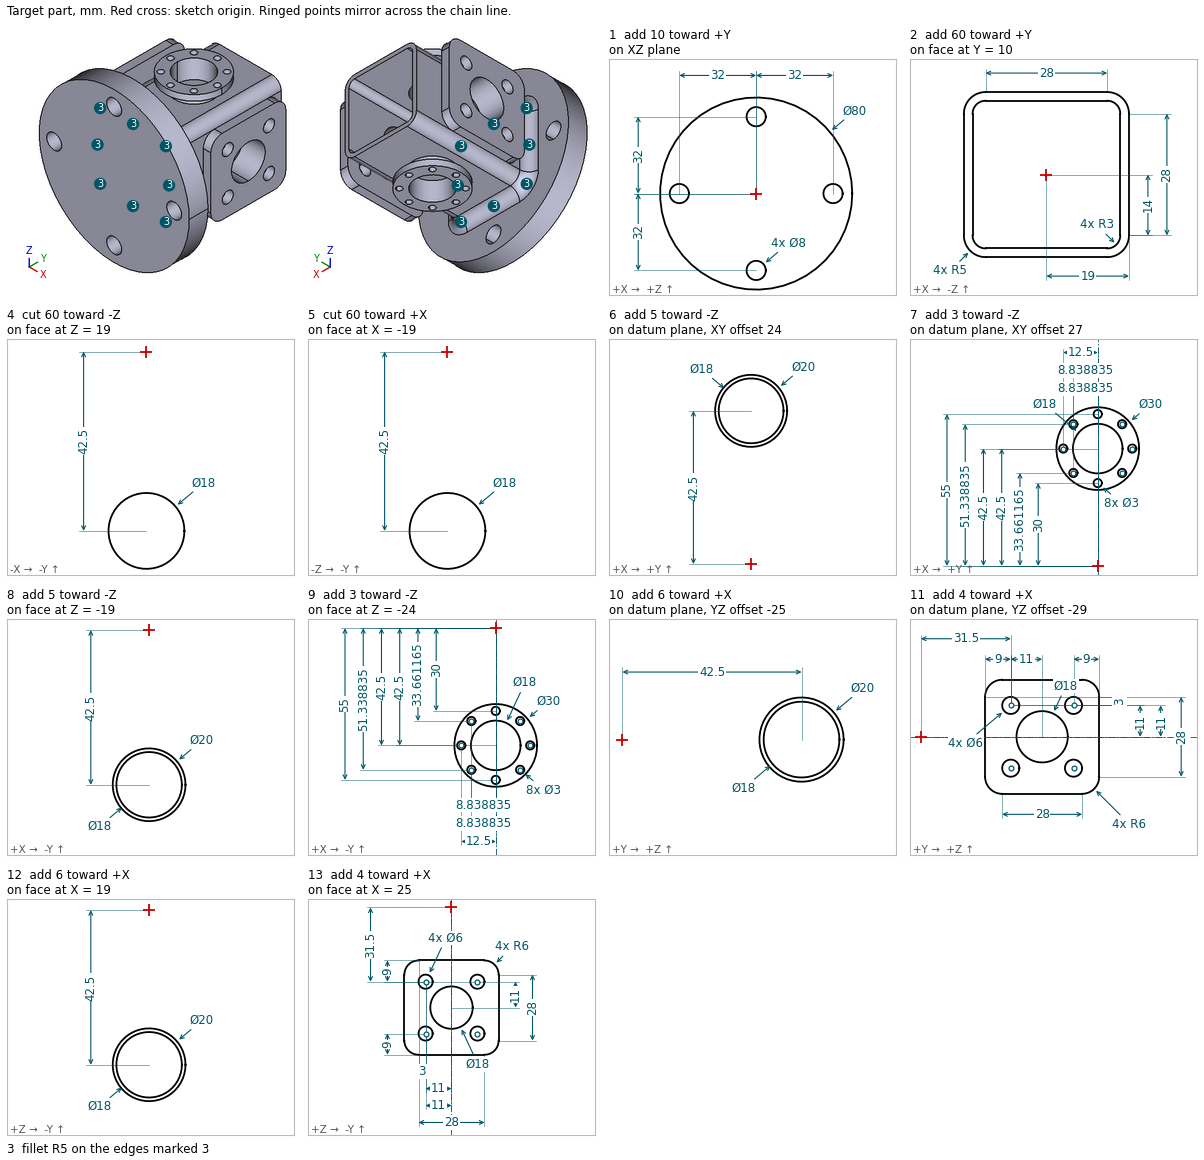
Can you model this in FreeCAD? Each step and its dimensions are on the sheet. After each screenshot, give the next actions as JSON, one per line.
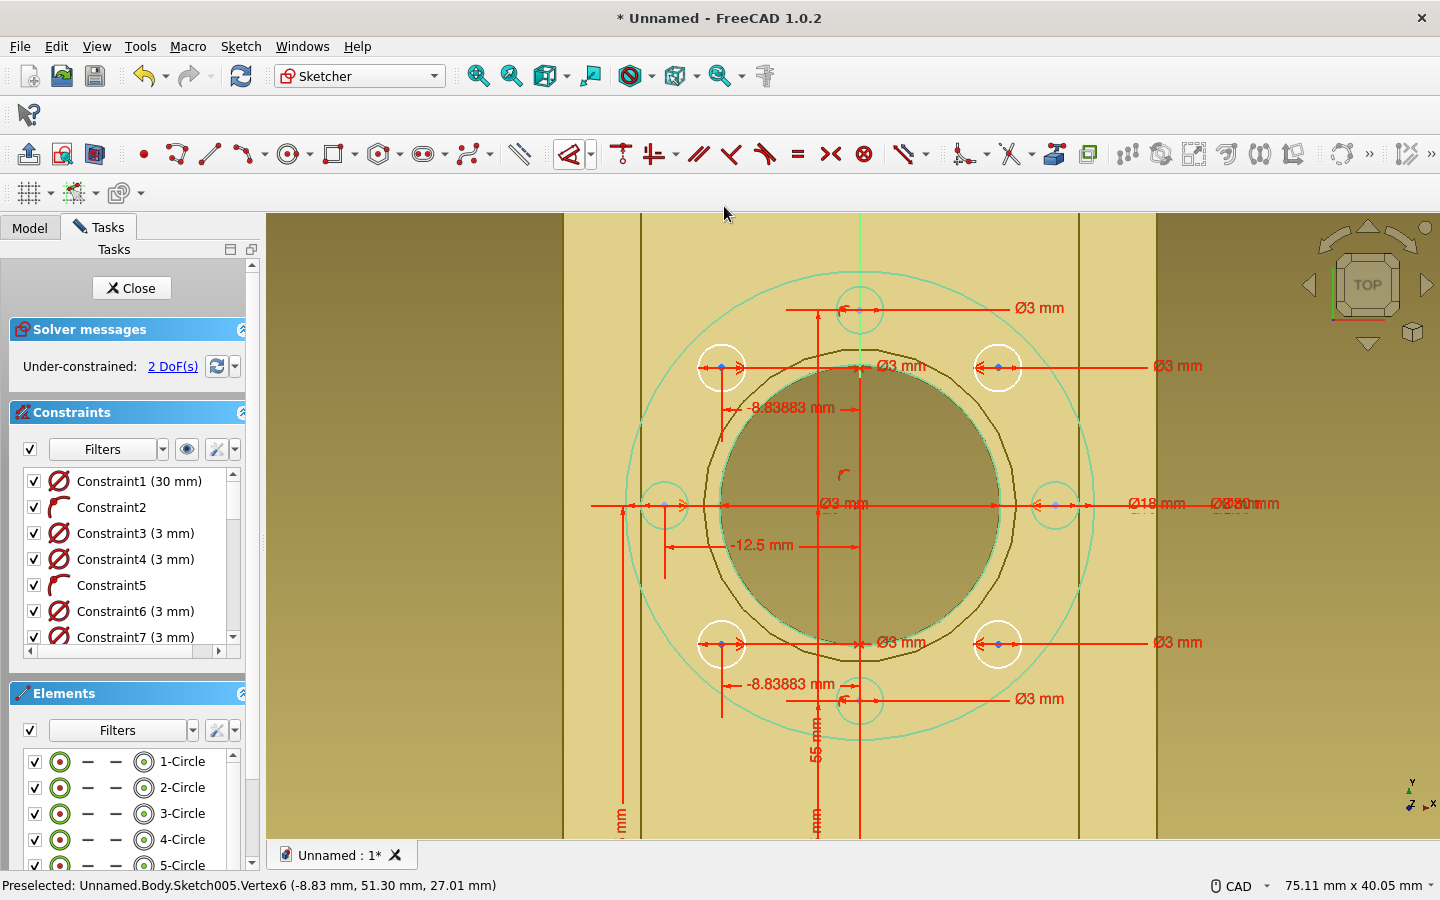
{"action": "left_click", "coordinate": [722, 644]}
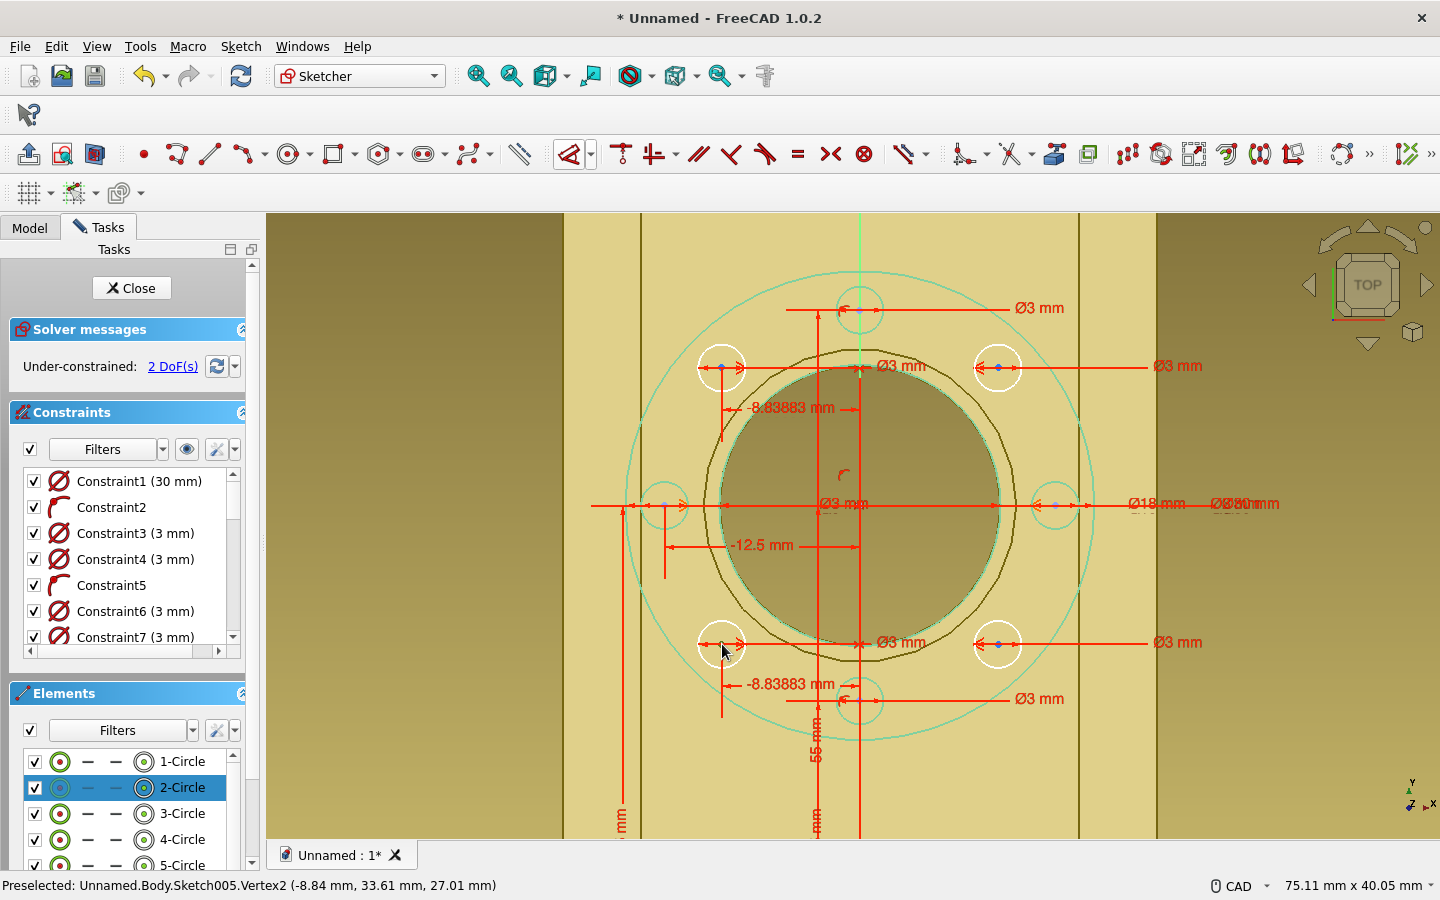
{"action": "left_click", "coordinate": [590, 154]}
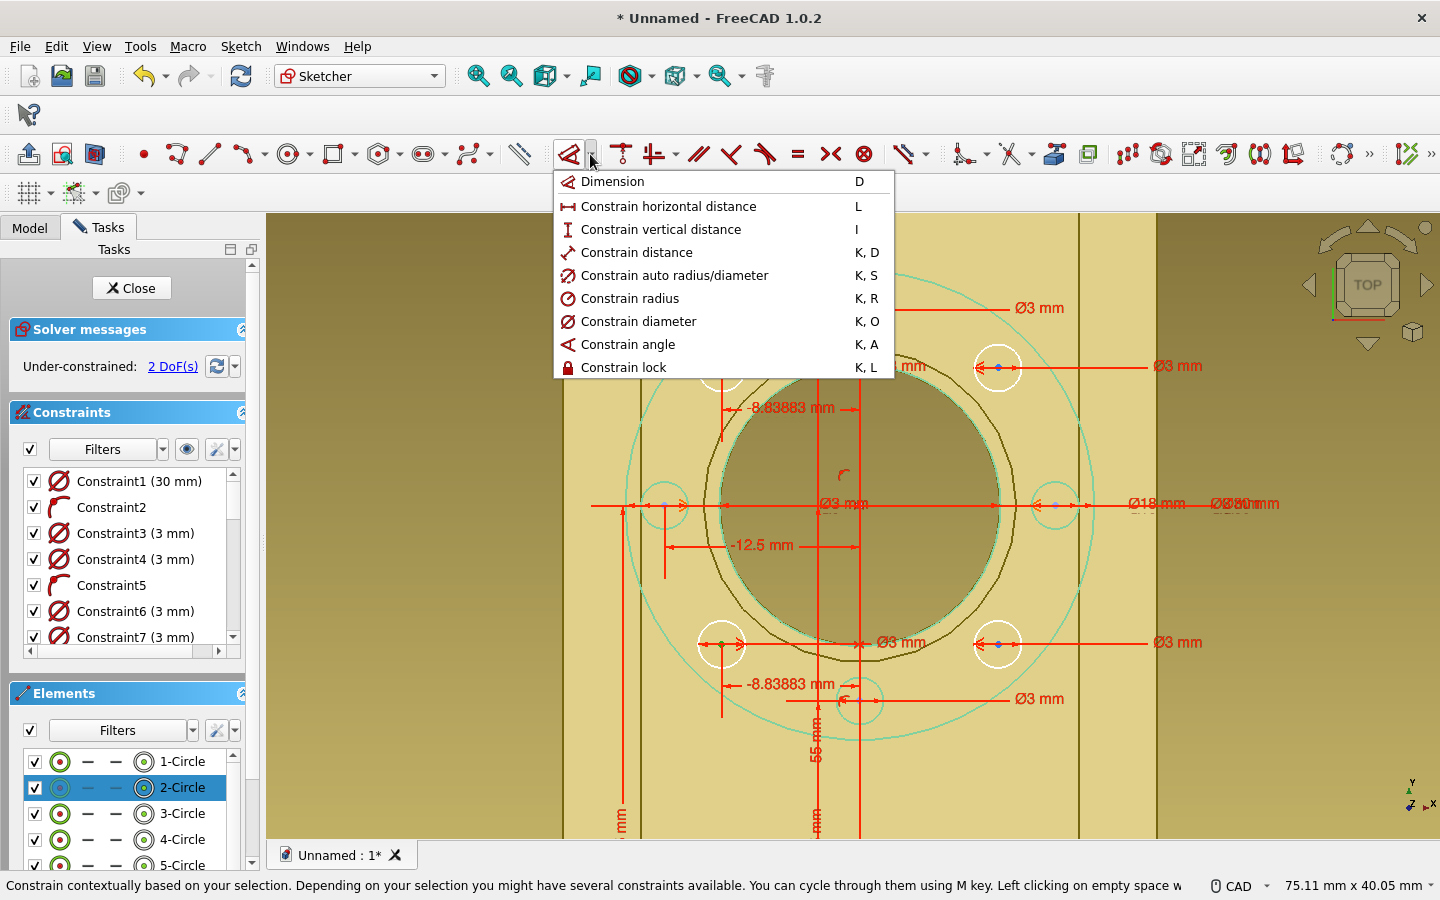
{"action": "left_click", "coordinate": [724, 230]}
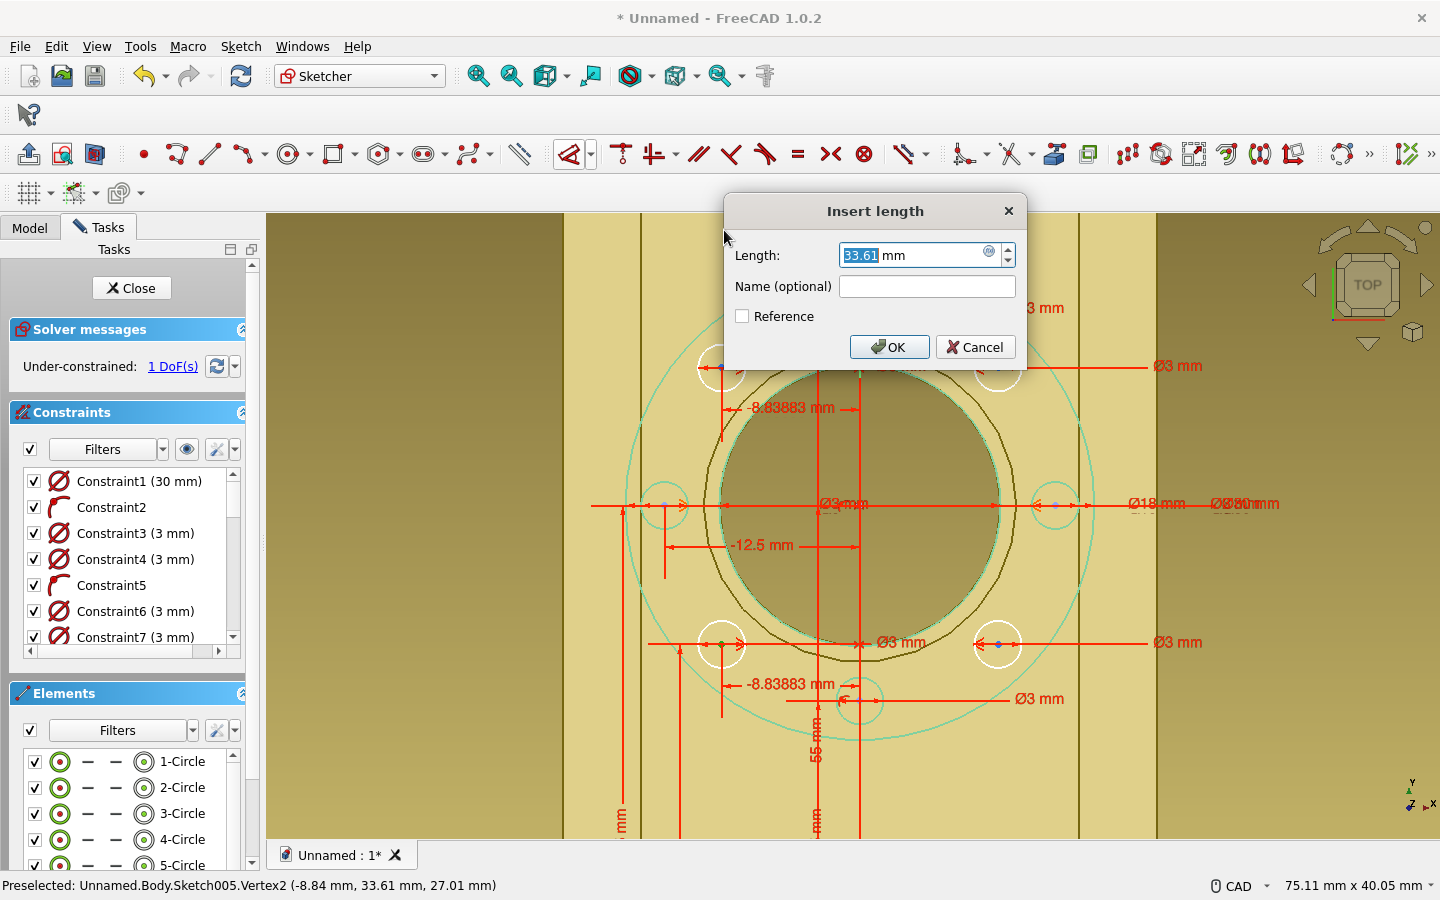
{"action": "type", "text": "33.661165"}
{"action": "key", "text": "Return"}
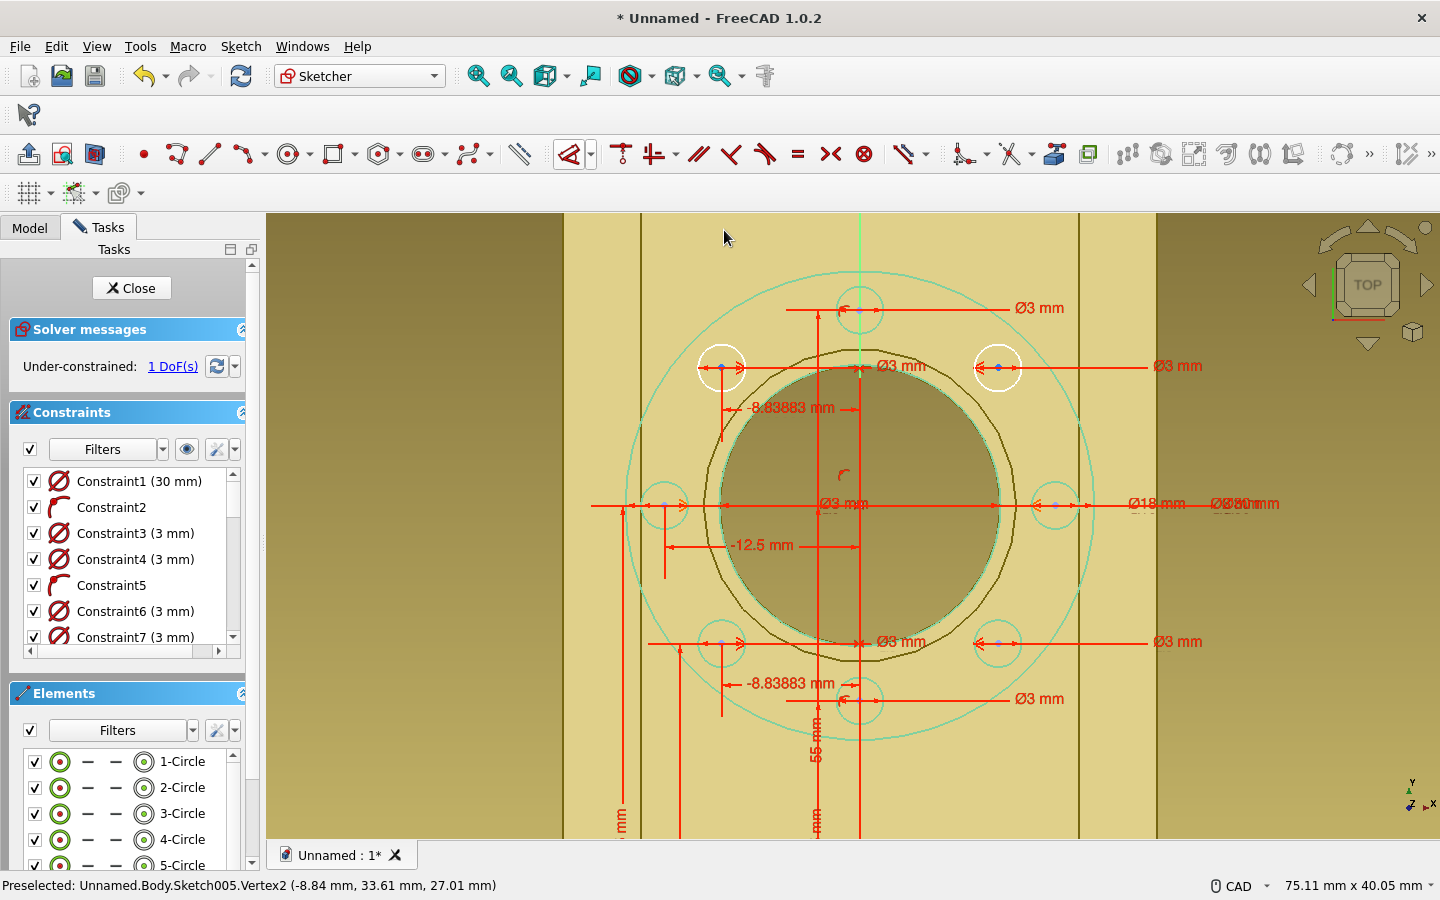
{"action": "left_click", "coordinate": [722, 368]}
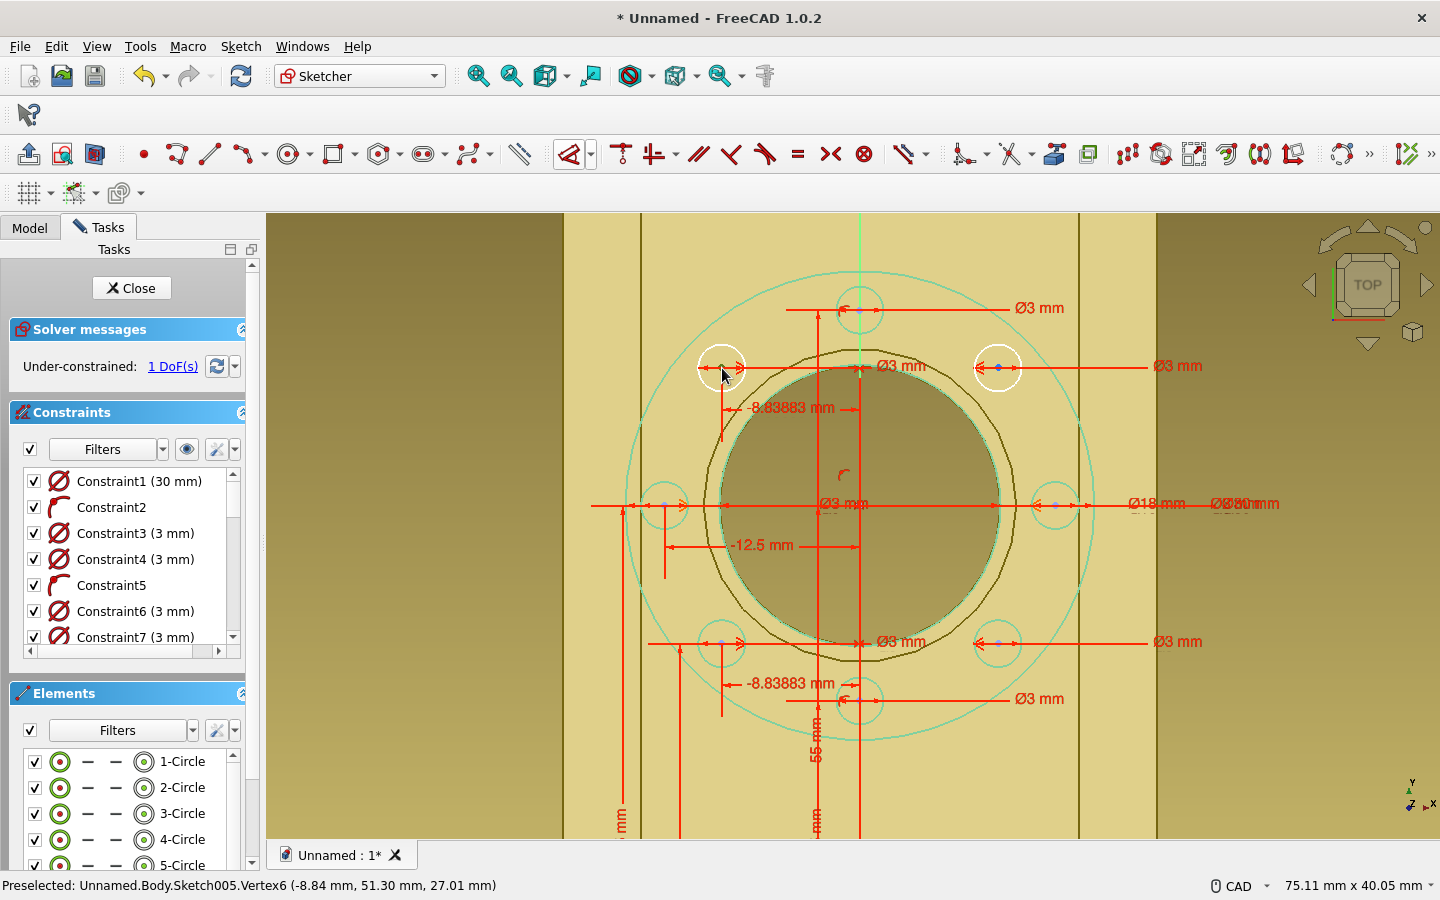
{"action": "key", "text": "i"}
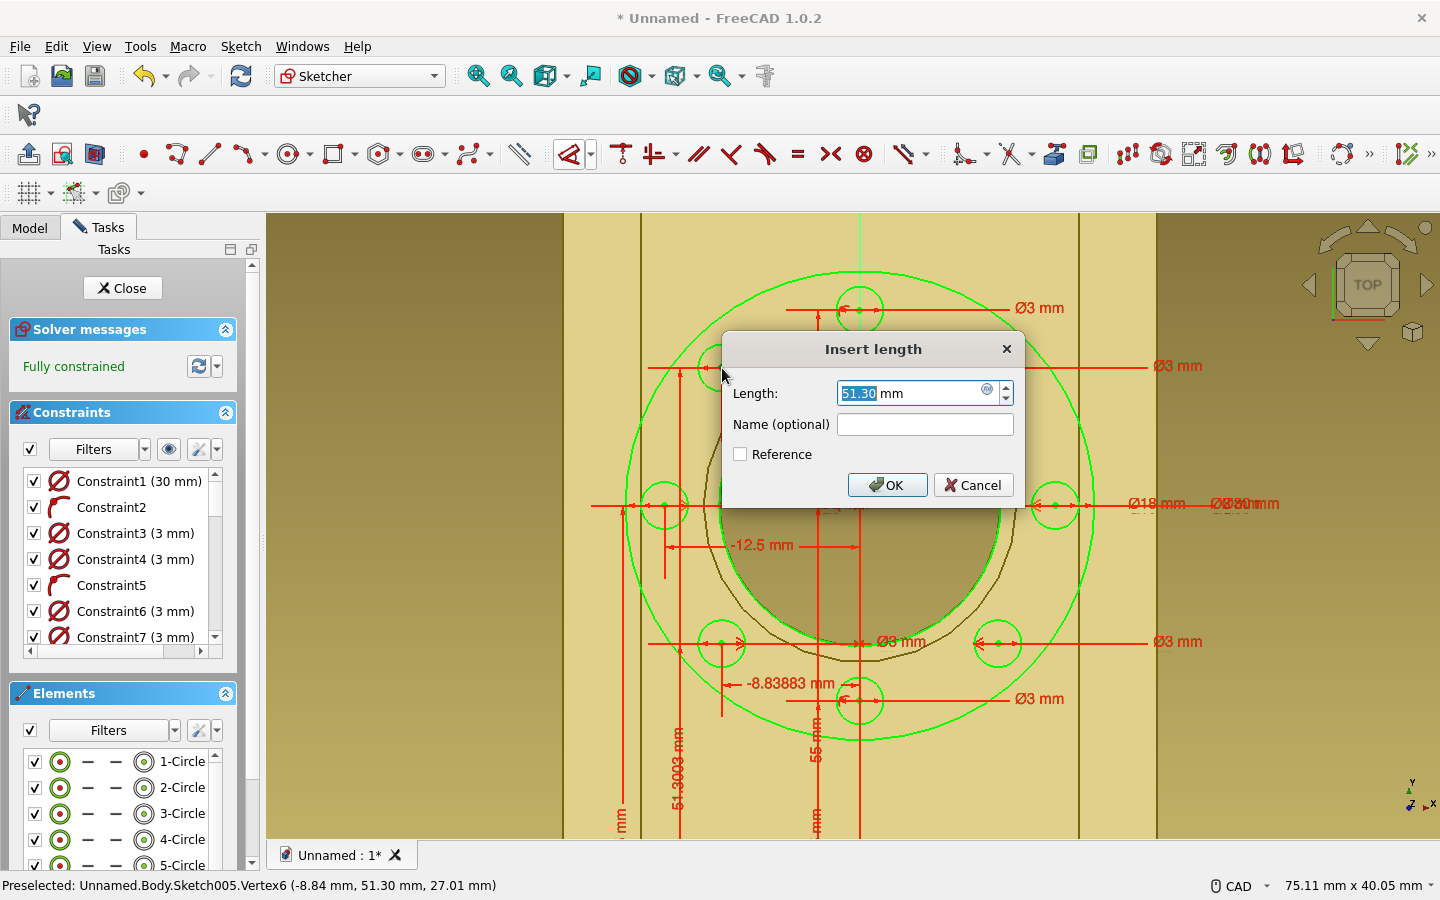
{"action": "type", "text": "51.338835"}
{"action": "key", "text": "Return"}